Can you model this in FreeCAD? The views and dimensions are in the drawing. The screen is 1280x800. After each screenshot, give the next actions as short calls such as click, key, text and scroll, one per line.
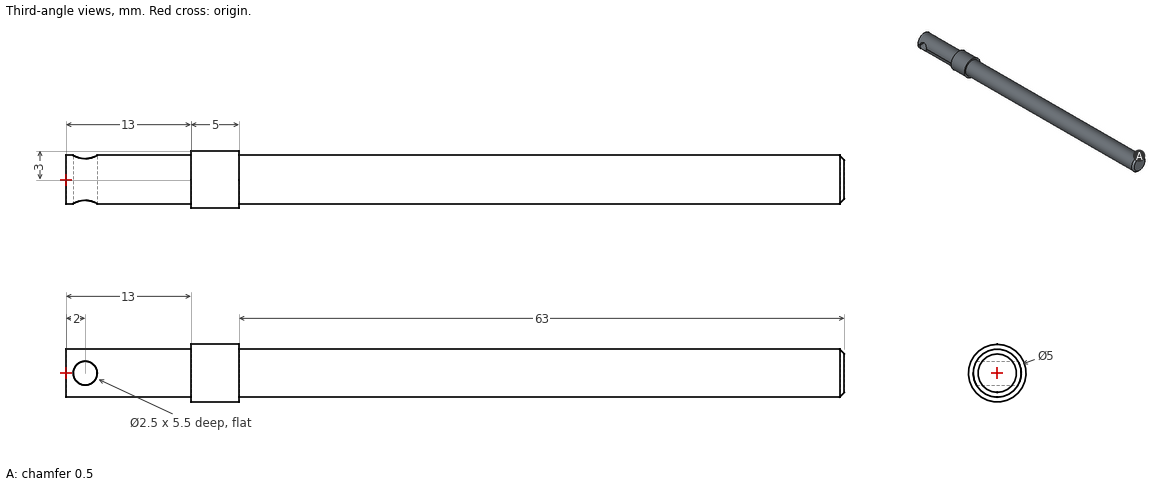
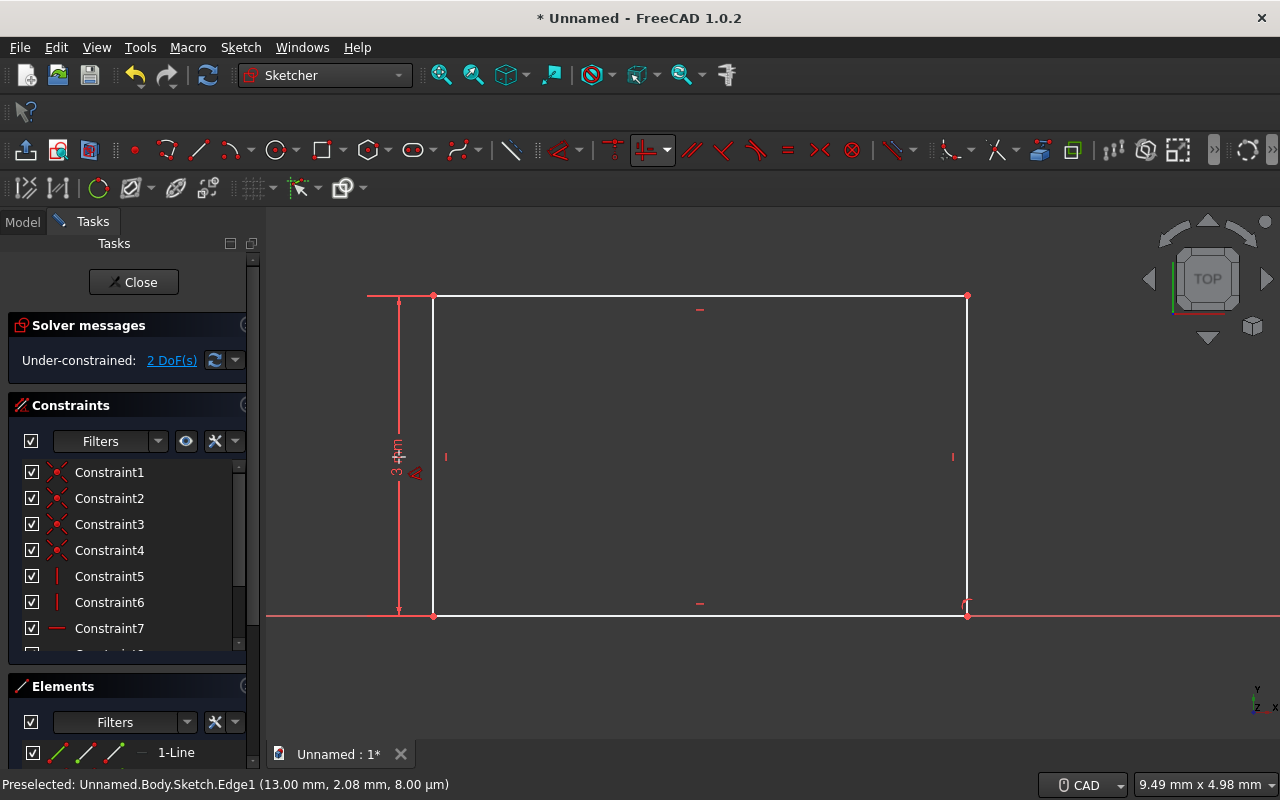
click(593, 616)
click(700, 650)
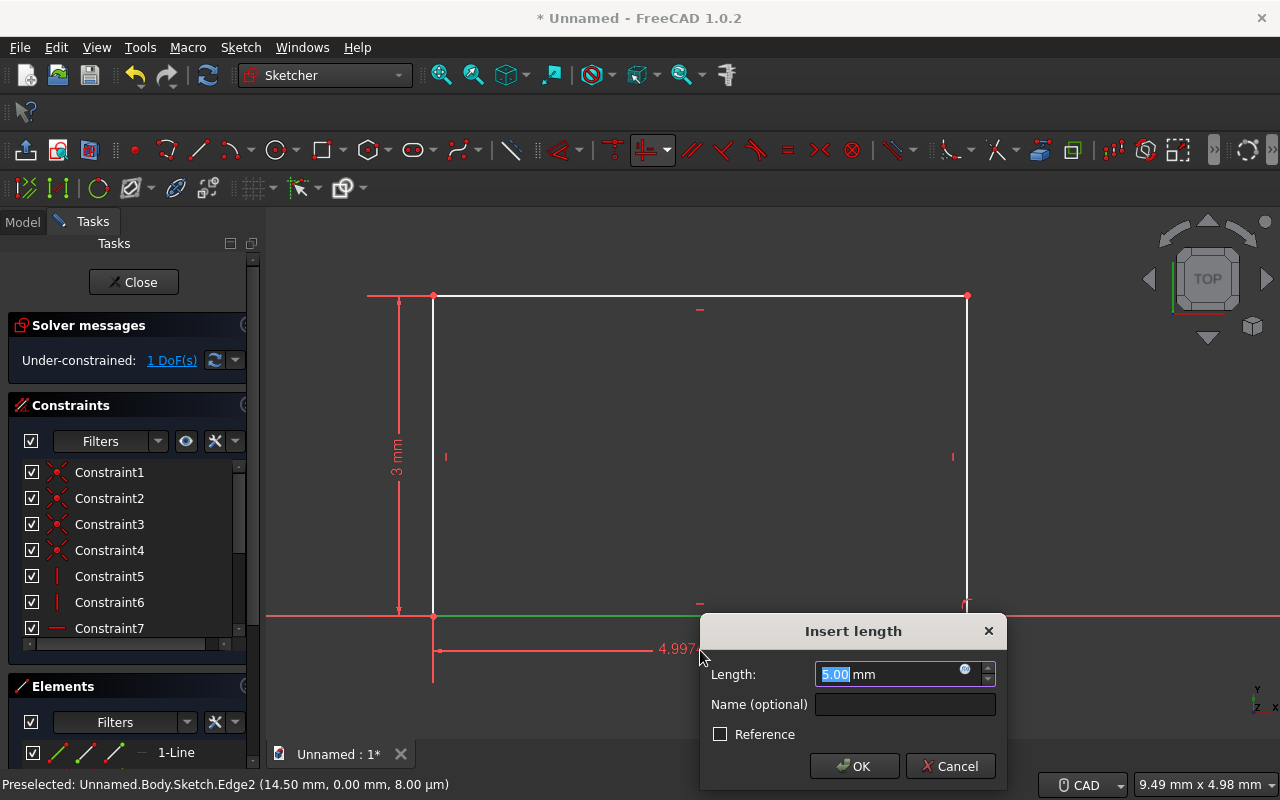
text(5)
key(Return)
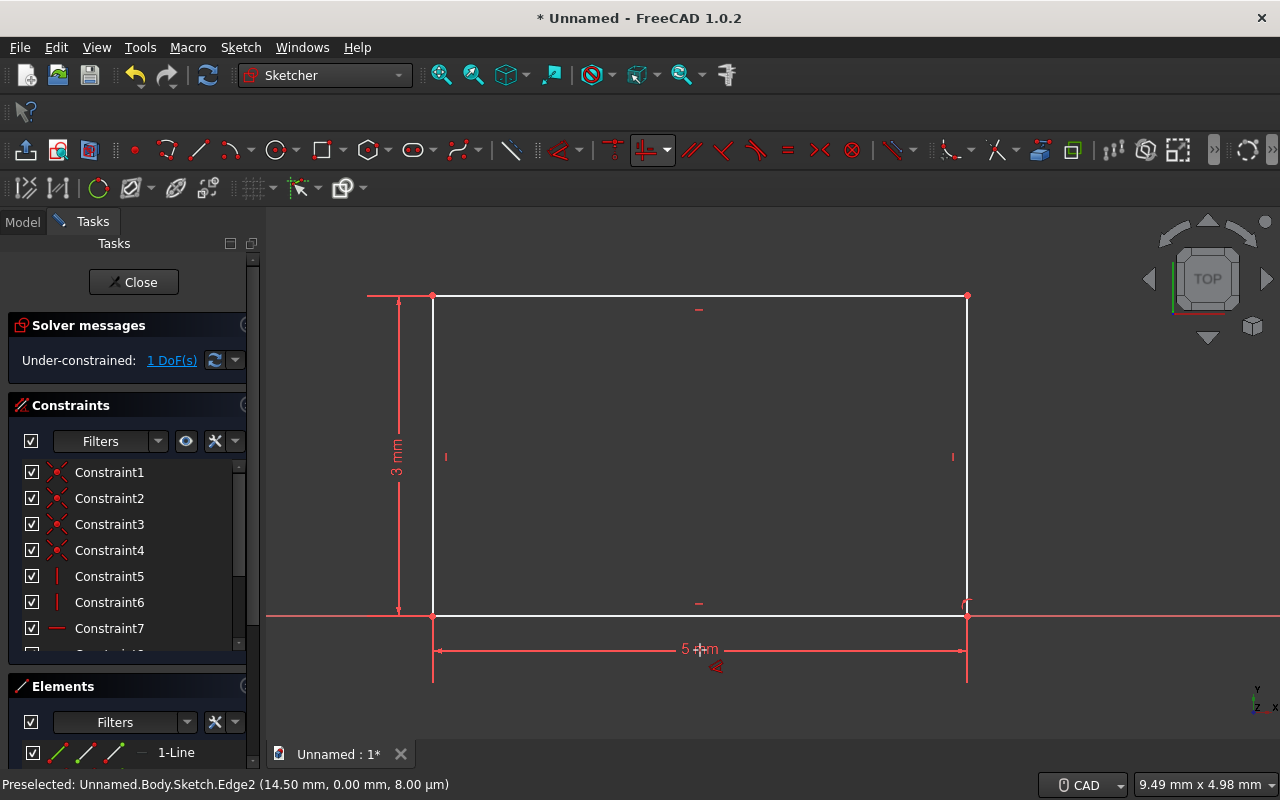
click(433, 296)
click(363, 650)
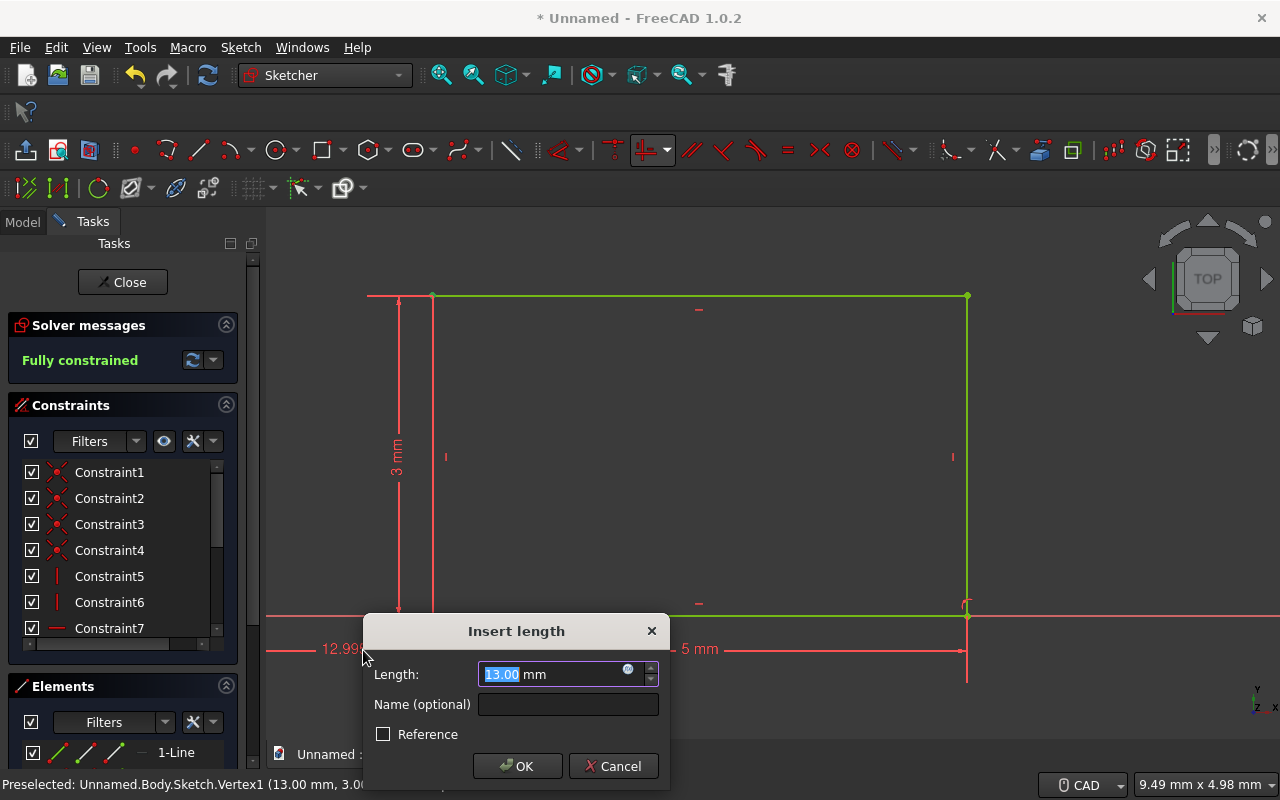
text(13)
key(Return)
key(Escape)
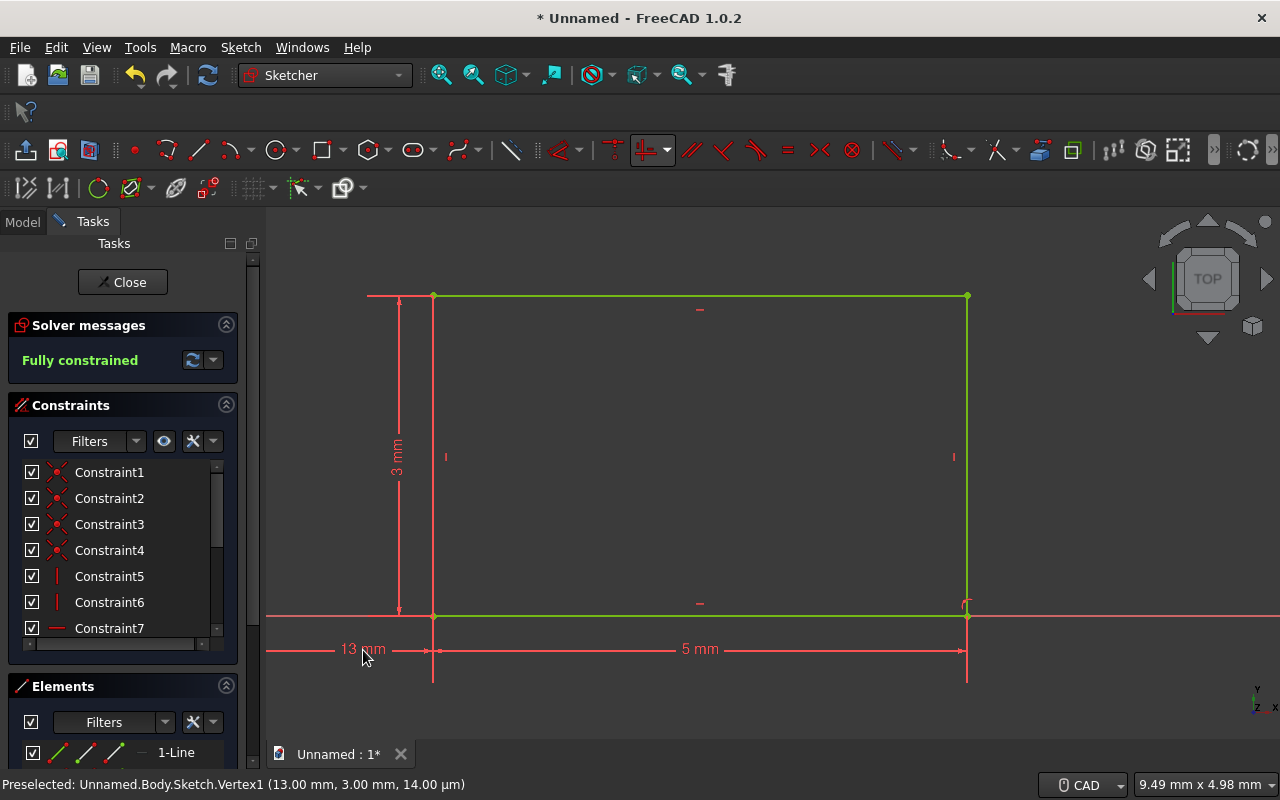
click(123, 282)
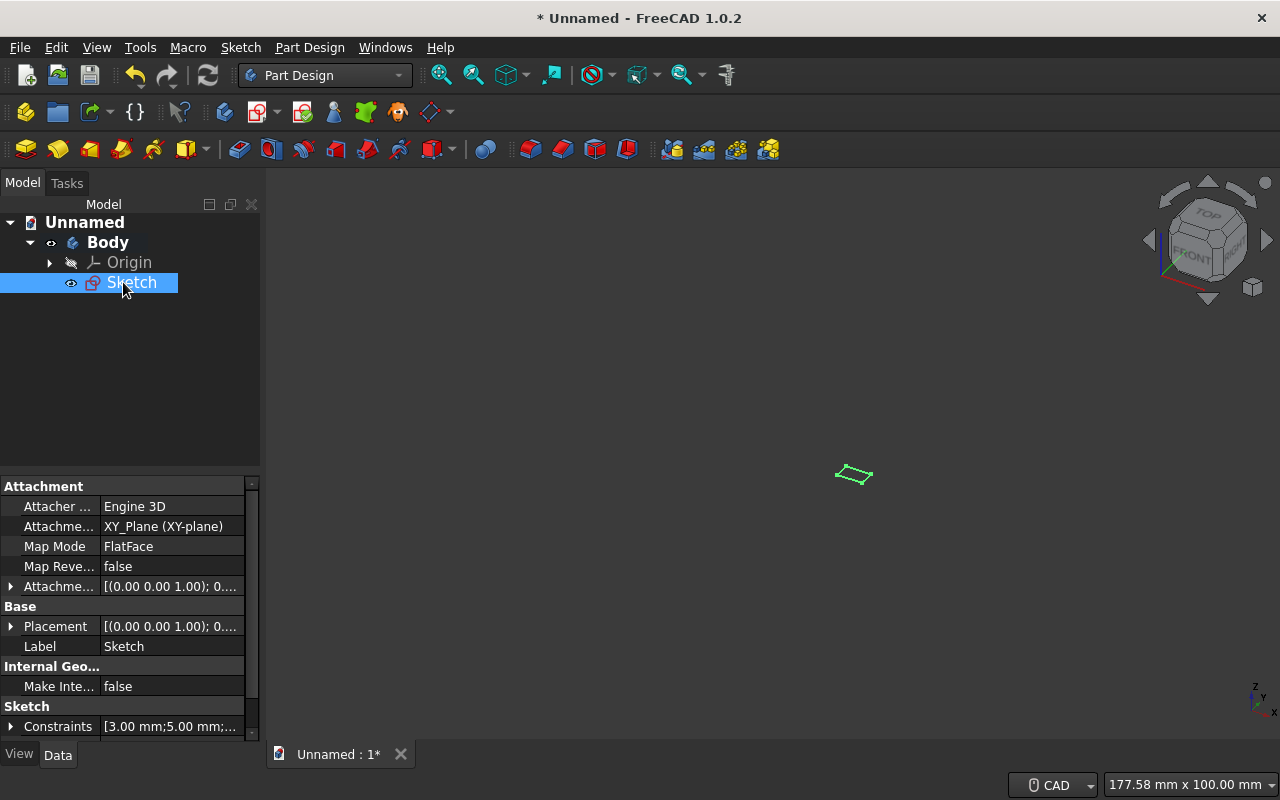
click(58, 150)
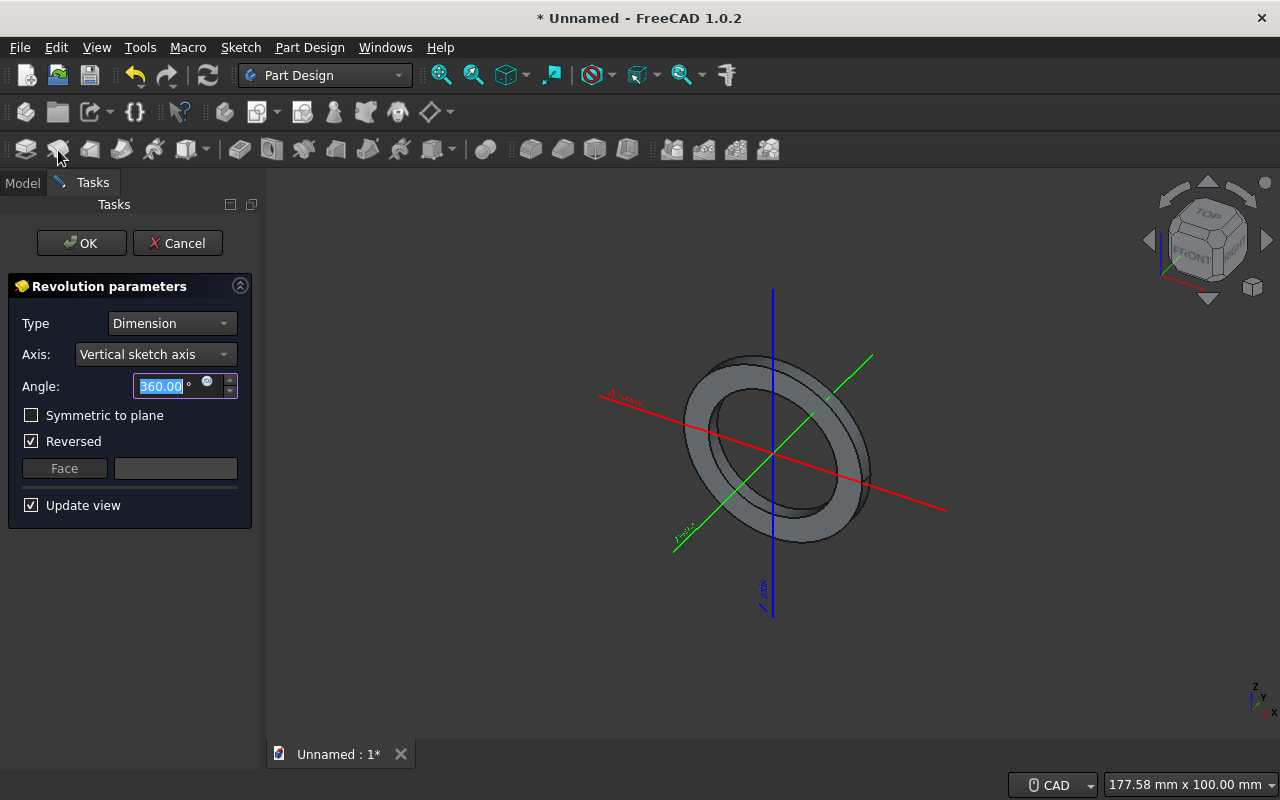
click(156, 354)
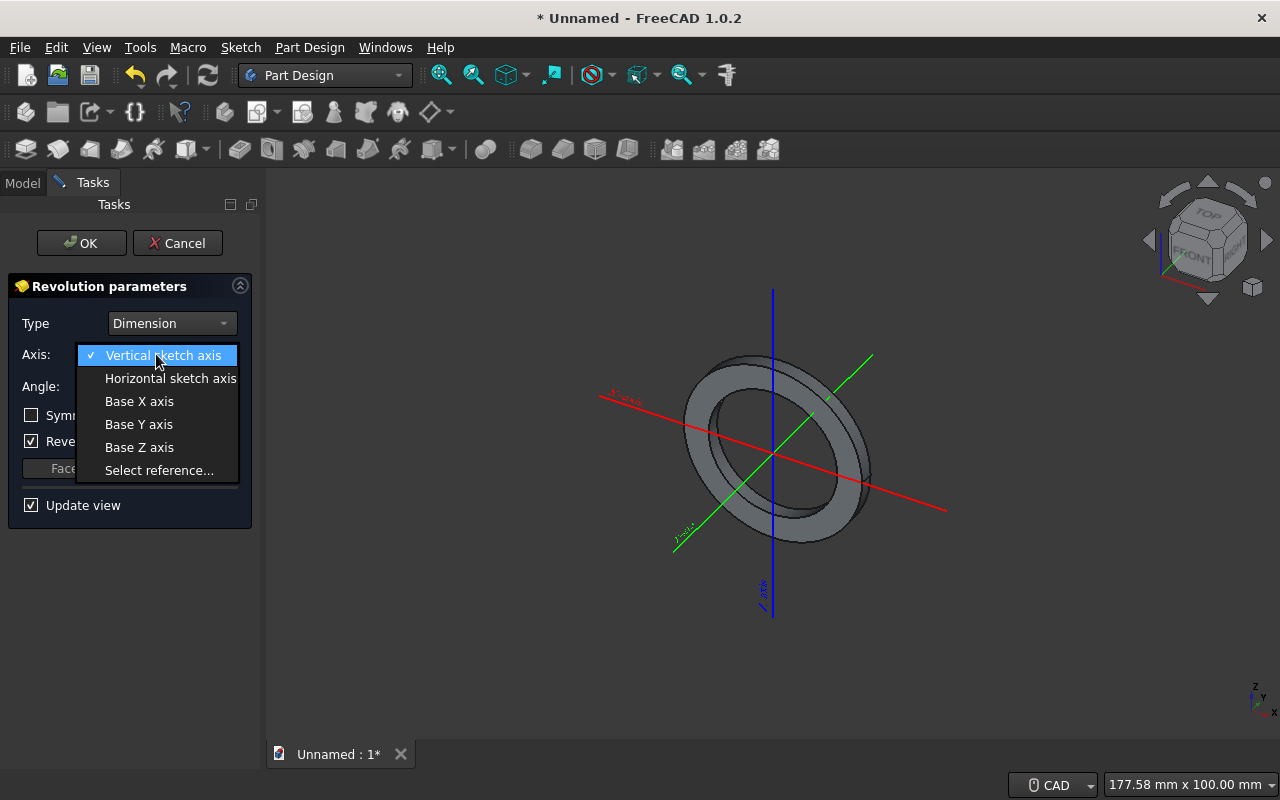
click(156, 378)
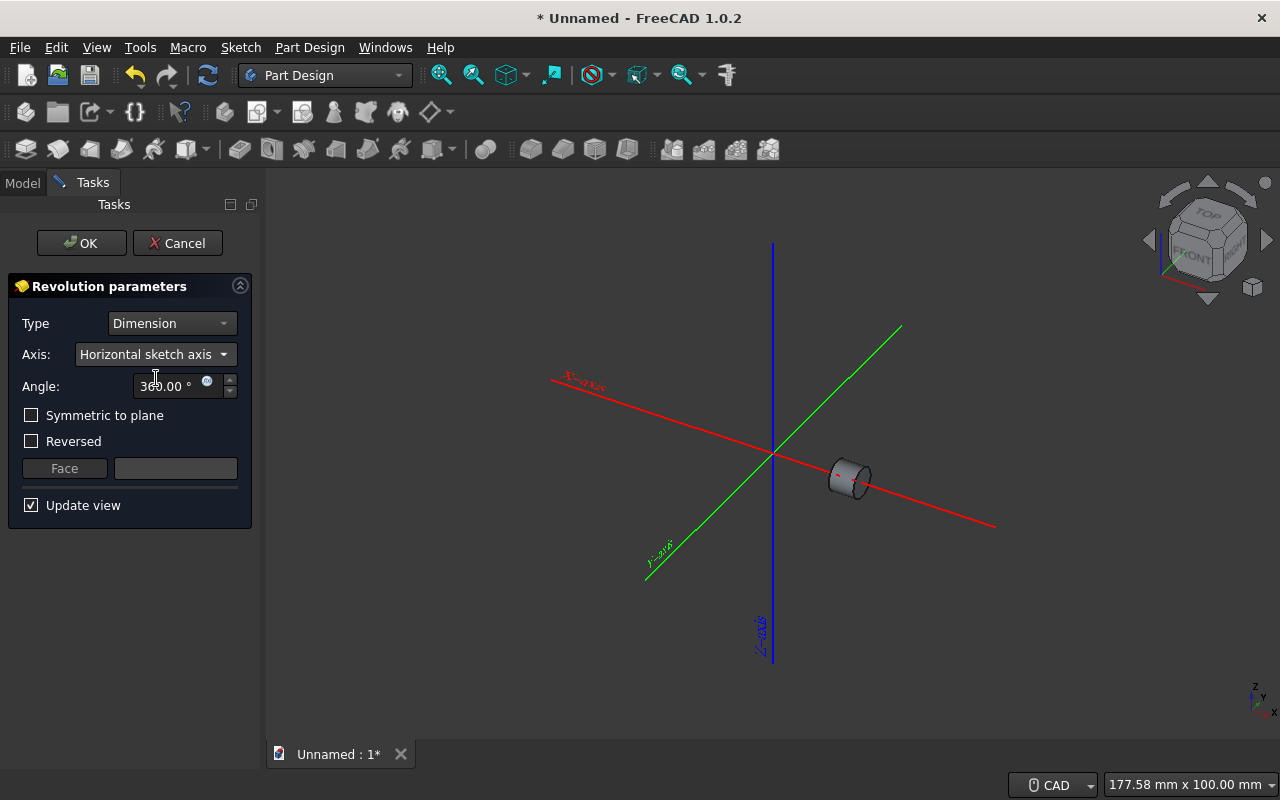
click(82, 243)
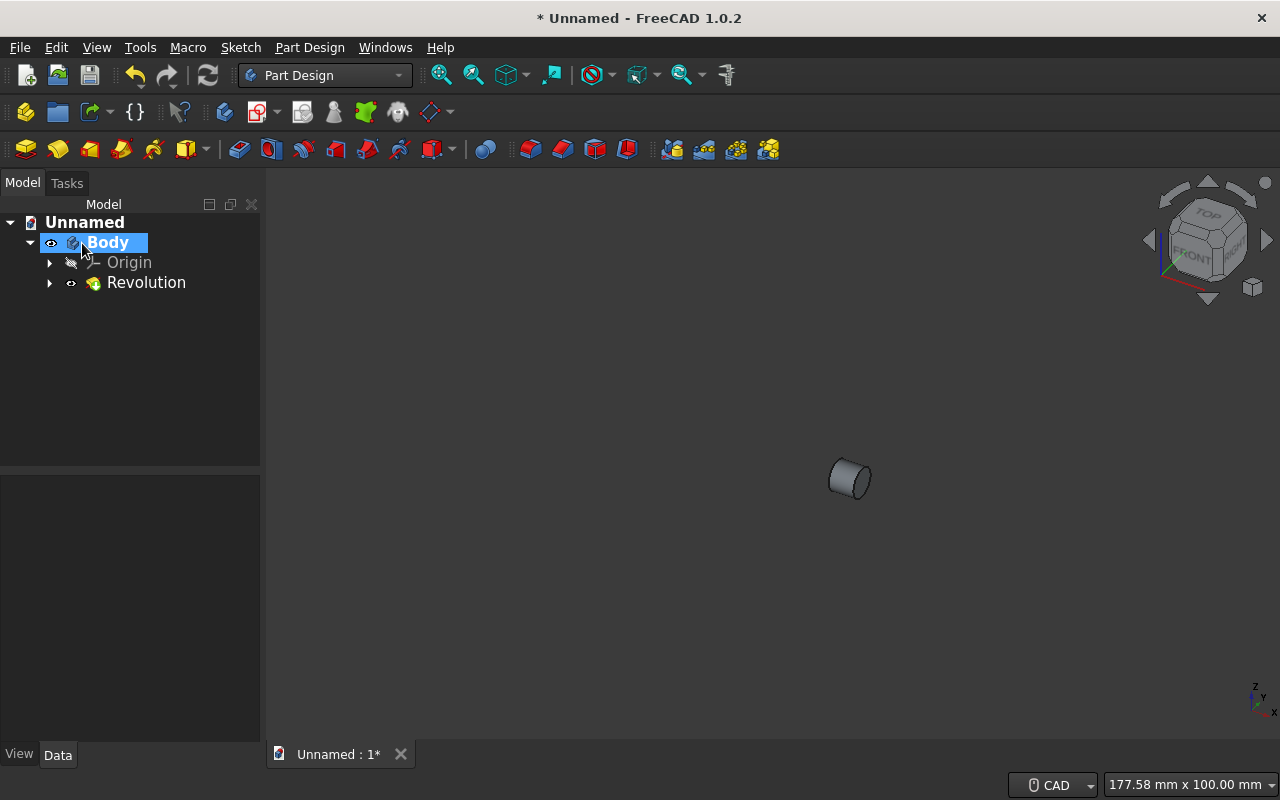
click(442, 76)